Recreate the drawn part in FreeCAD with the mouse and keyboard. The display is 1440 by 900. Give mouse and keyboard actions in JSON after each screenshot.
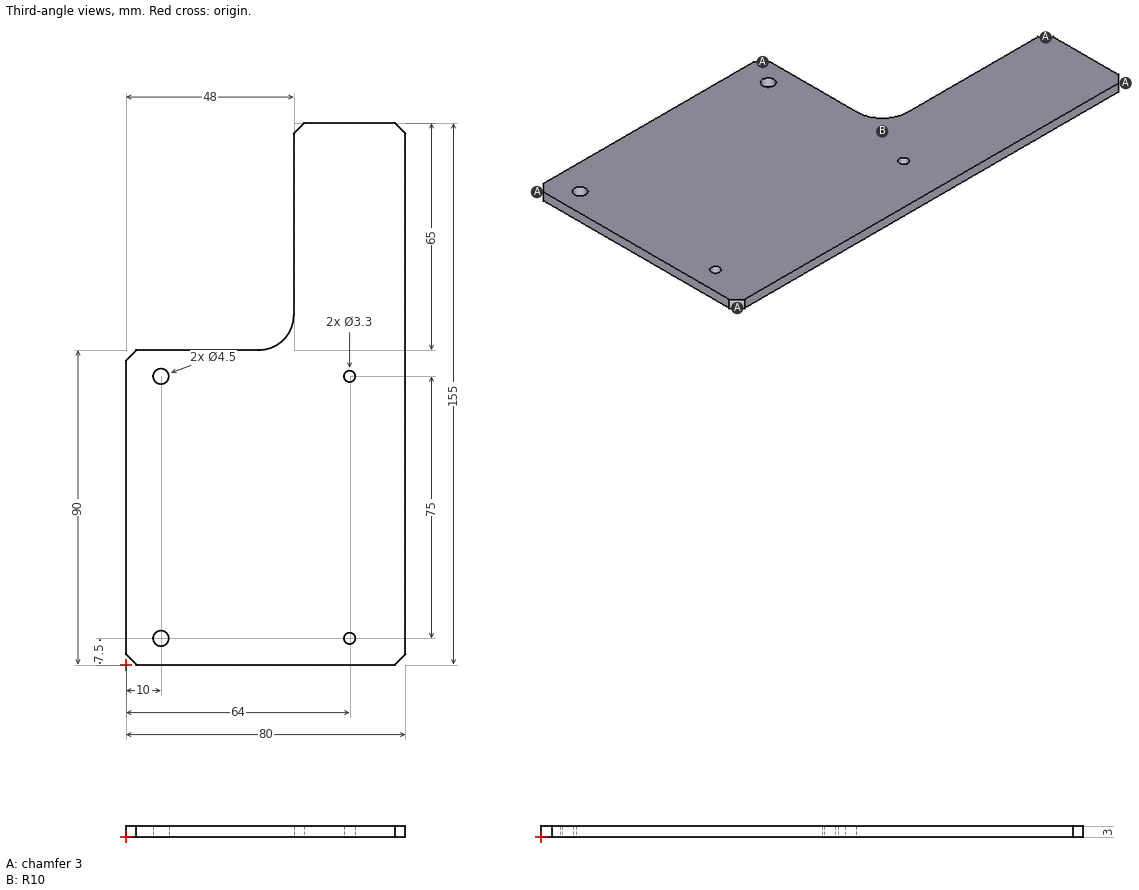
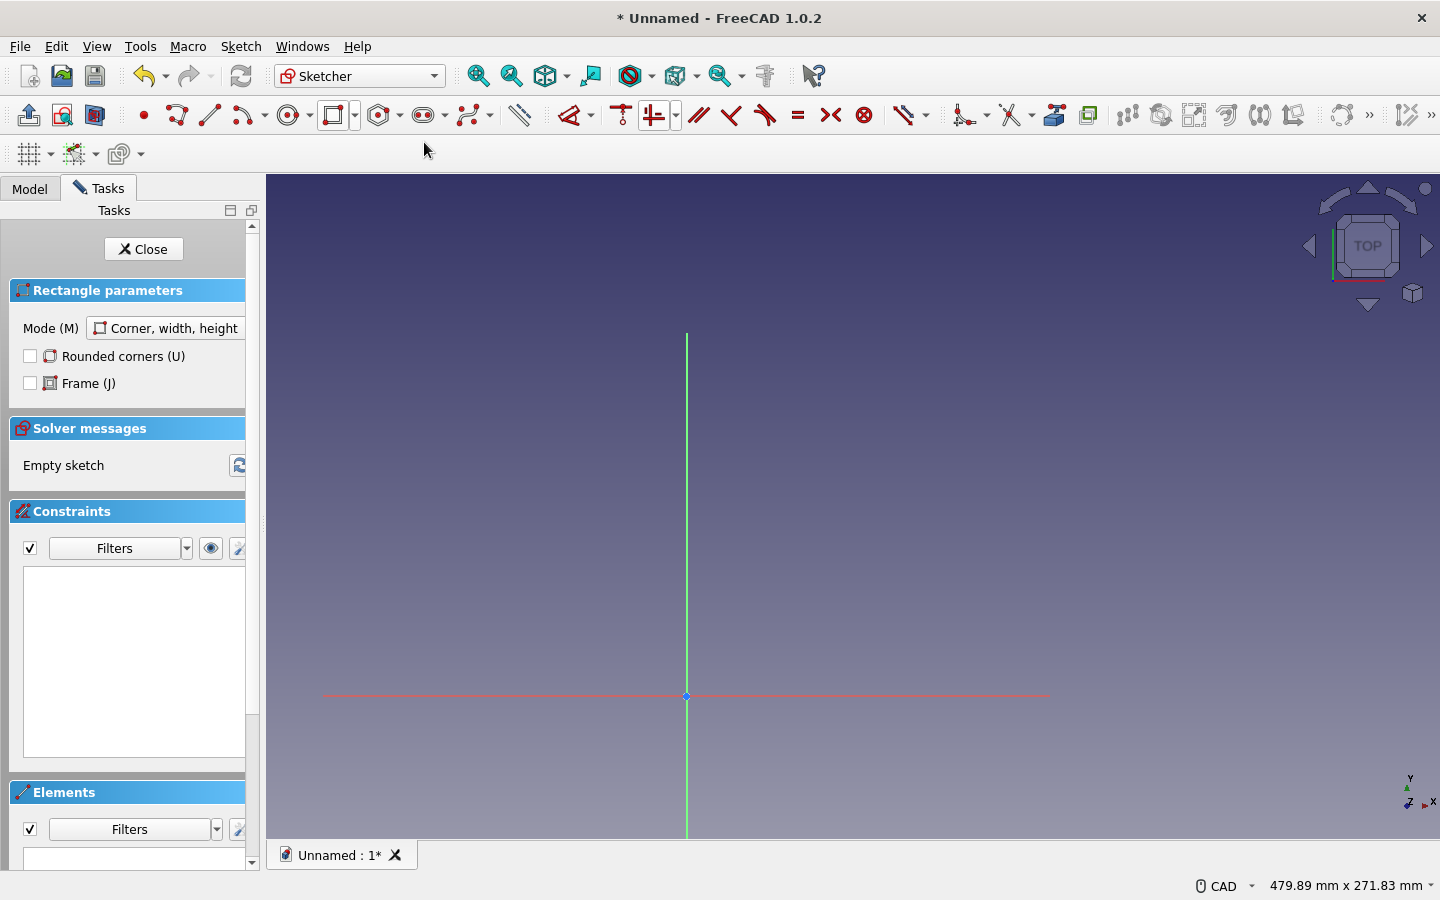
{"action": "left_click", "coordinate": [687, 696]}
{"action": "mouse_move", "coordinate": [883, 317]}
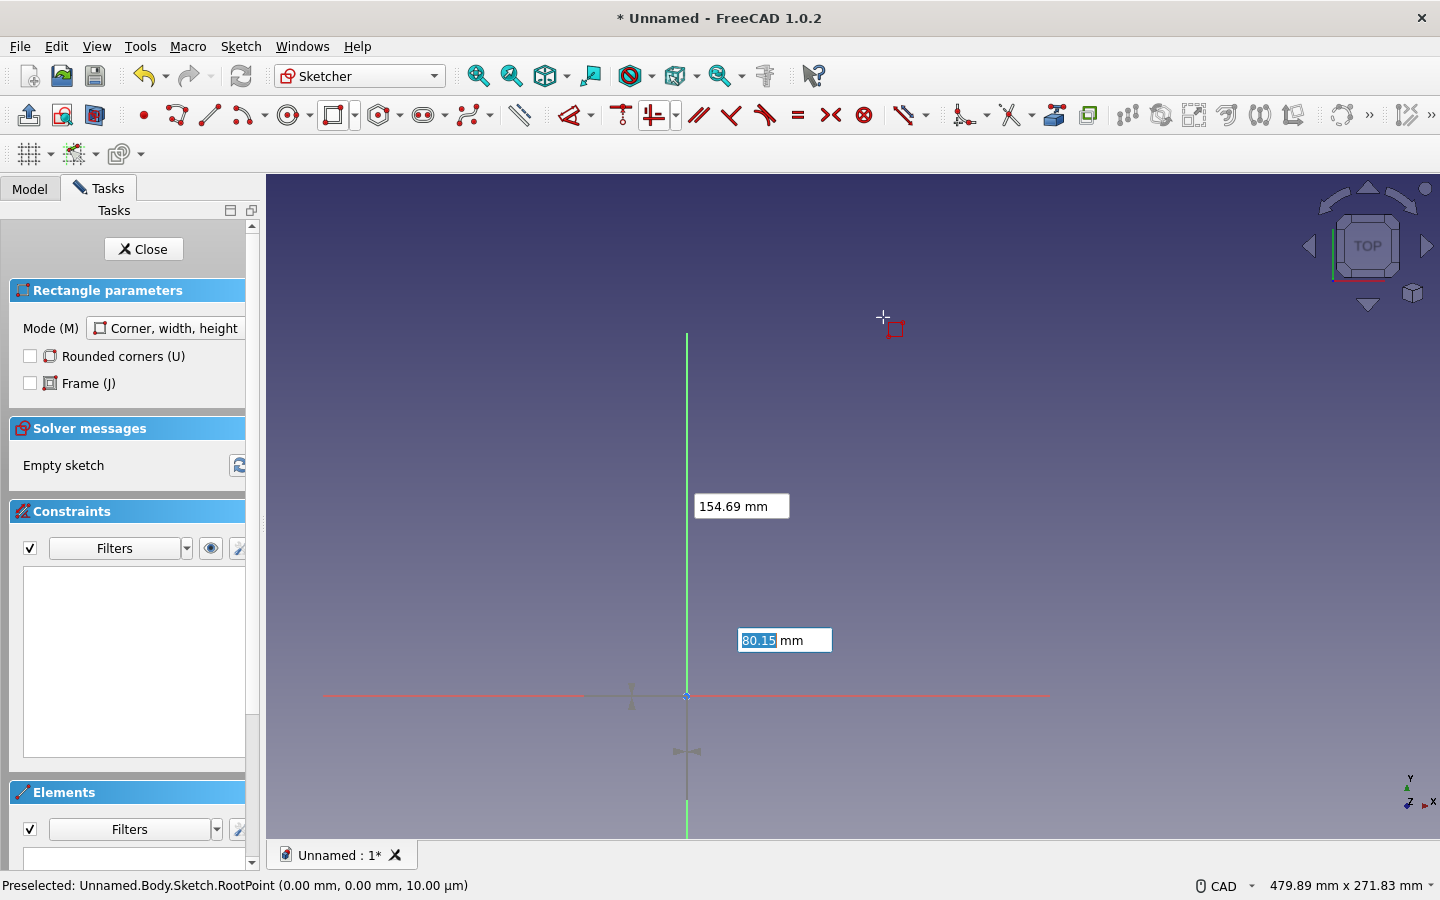
{"action": "type", "text": "80"}
{"action": "key", "text": "Tab"}
{"action": "type", "text": "155"}
{"action": "key", "text": "Return"}
{"action": "key", "text": "Escape"}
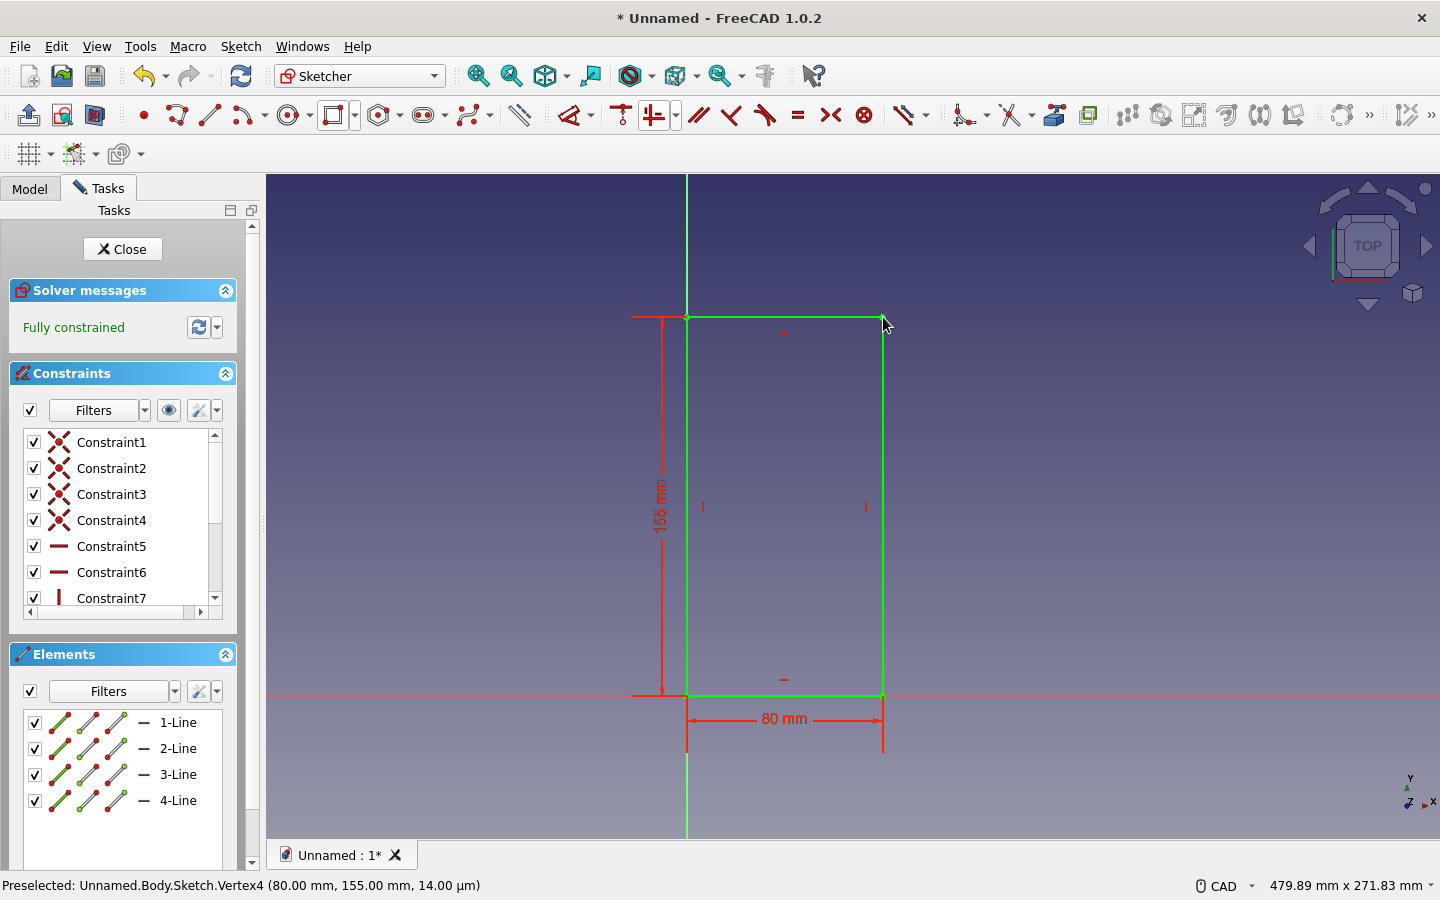
{"action": "left_click", "coordinate": [123, 249]}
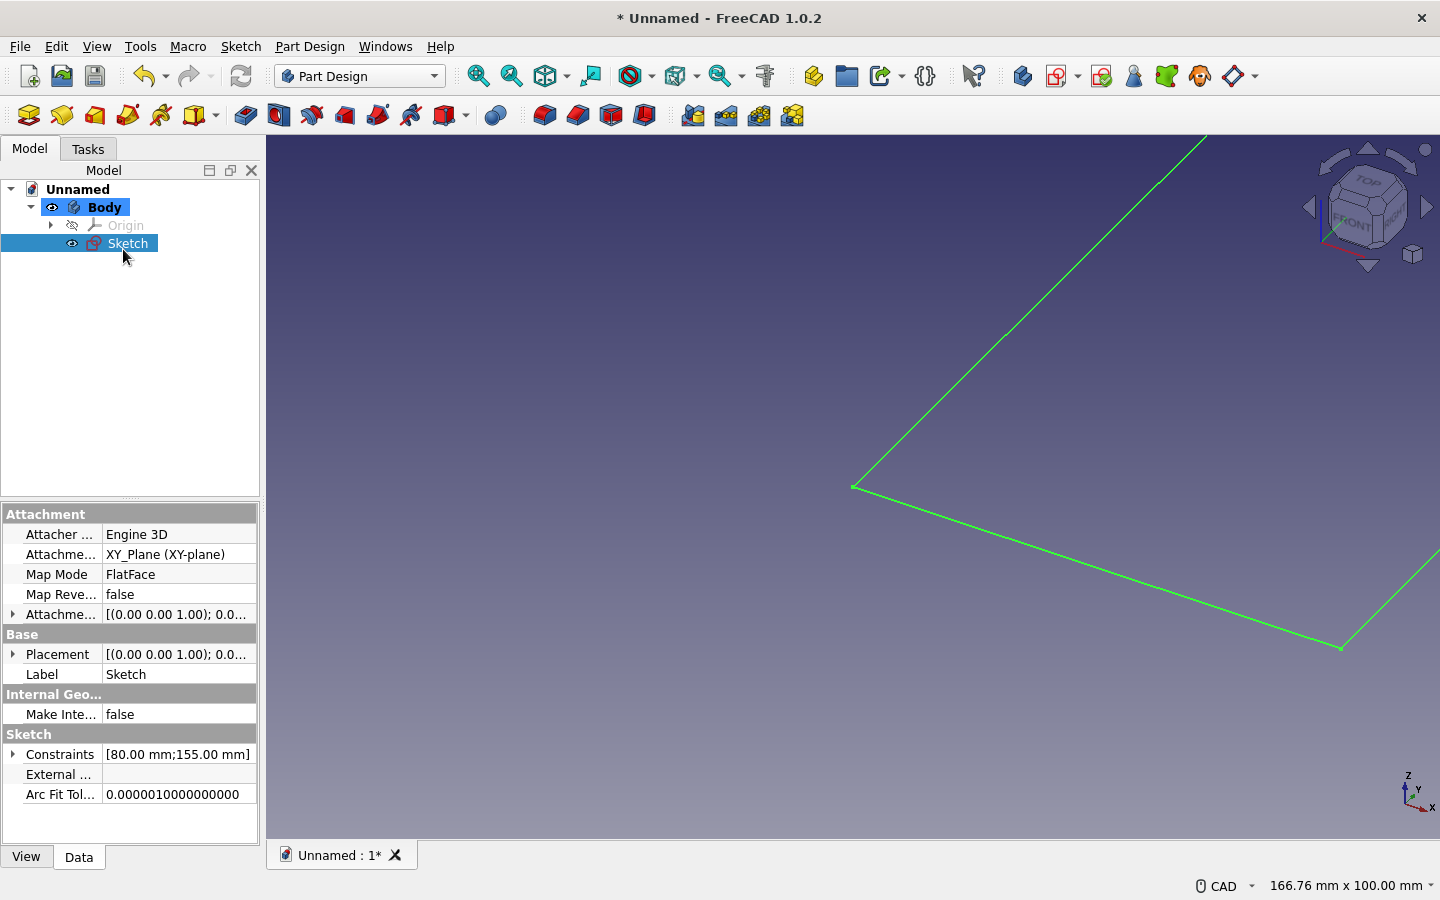
{"action": "left_click", "coordinate": [29, 116]}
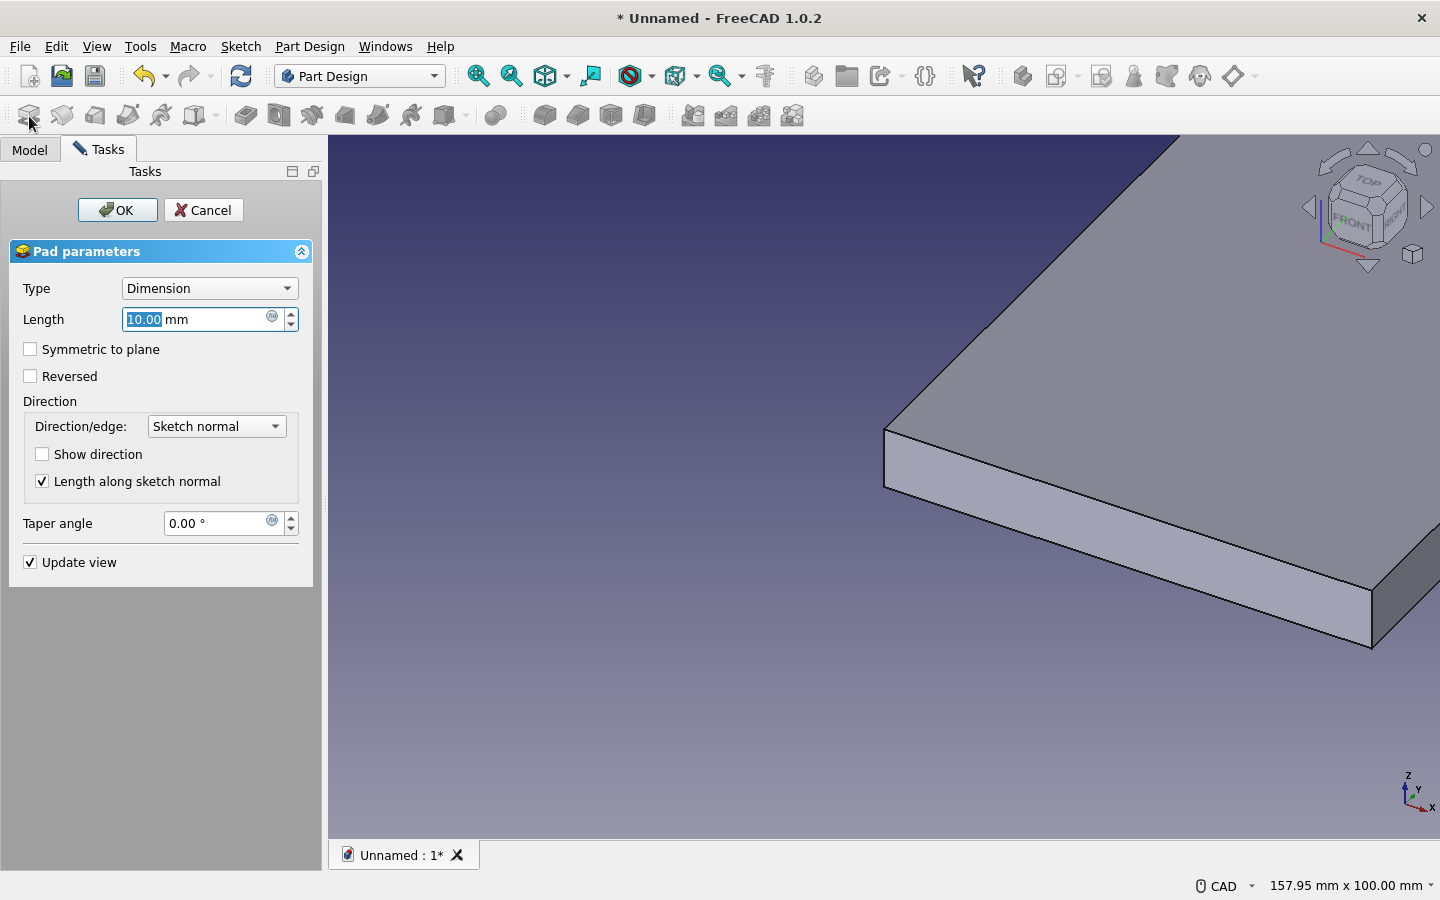
{"action": "type", "text": "3"}
{"action": "key", "text": "Tab"}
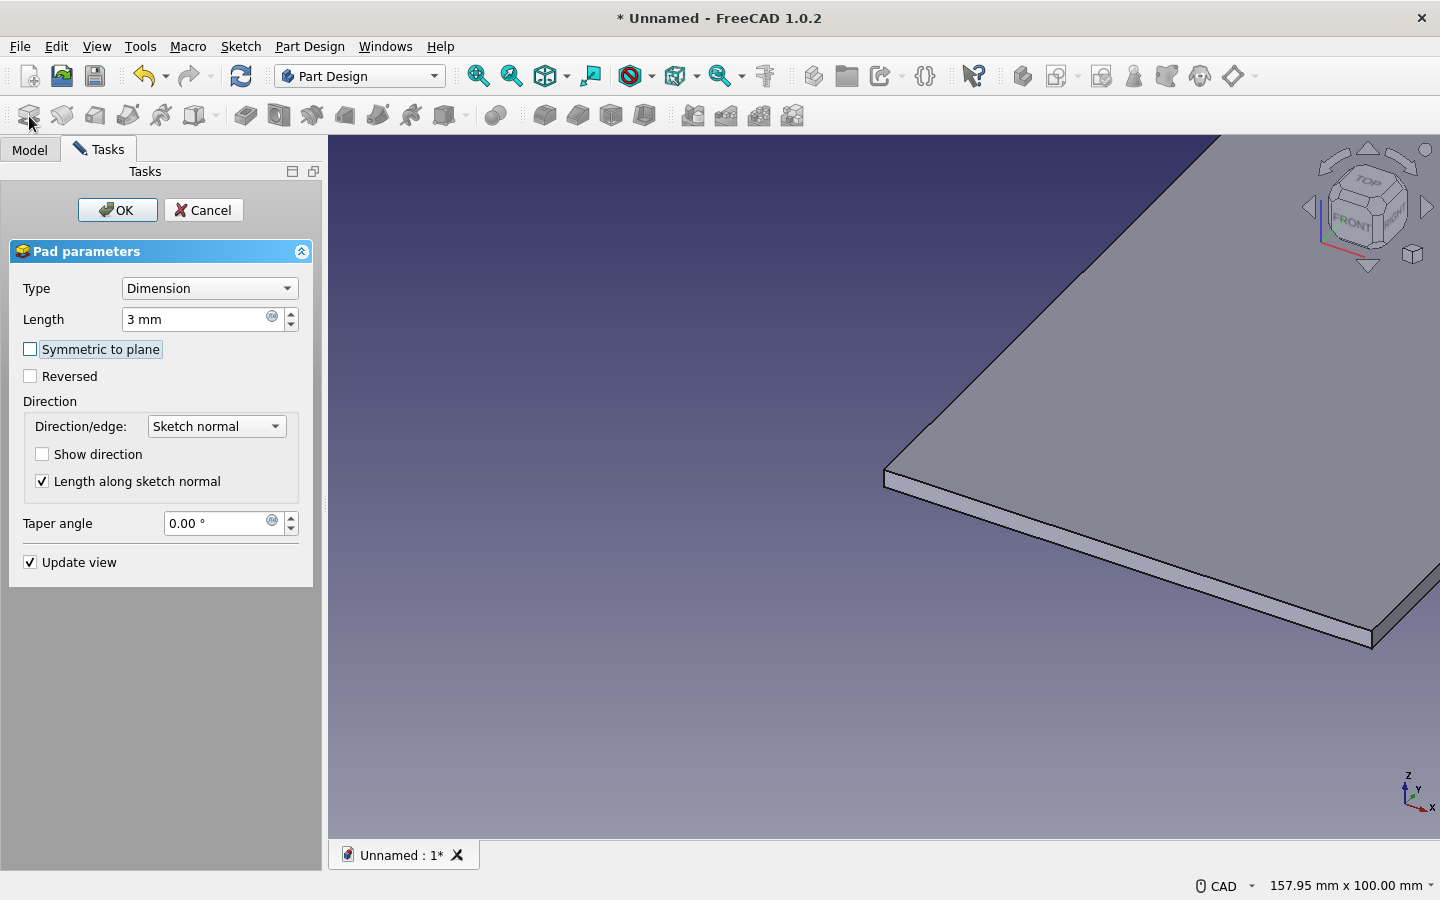
{"action": "left_click", "coordinate": [118, 210]}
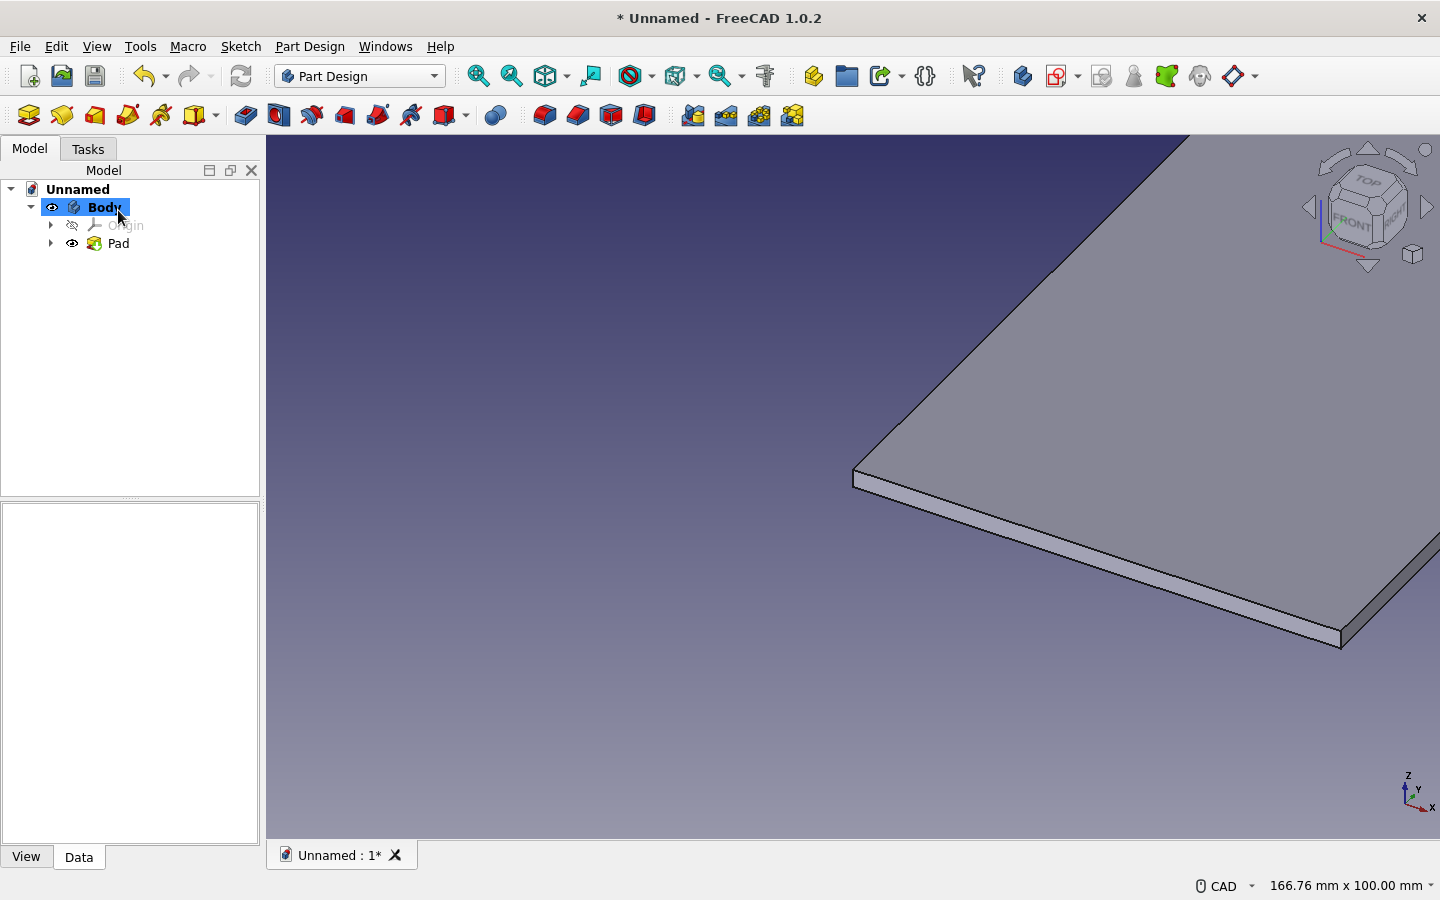
{"action": "key", "text": "v f"}